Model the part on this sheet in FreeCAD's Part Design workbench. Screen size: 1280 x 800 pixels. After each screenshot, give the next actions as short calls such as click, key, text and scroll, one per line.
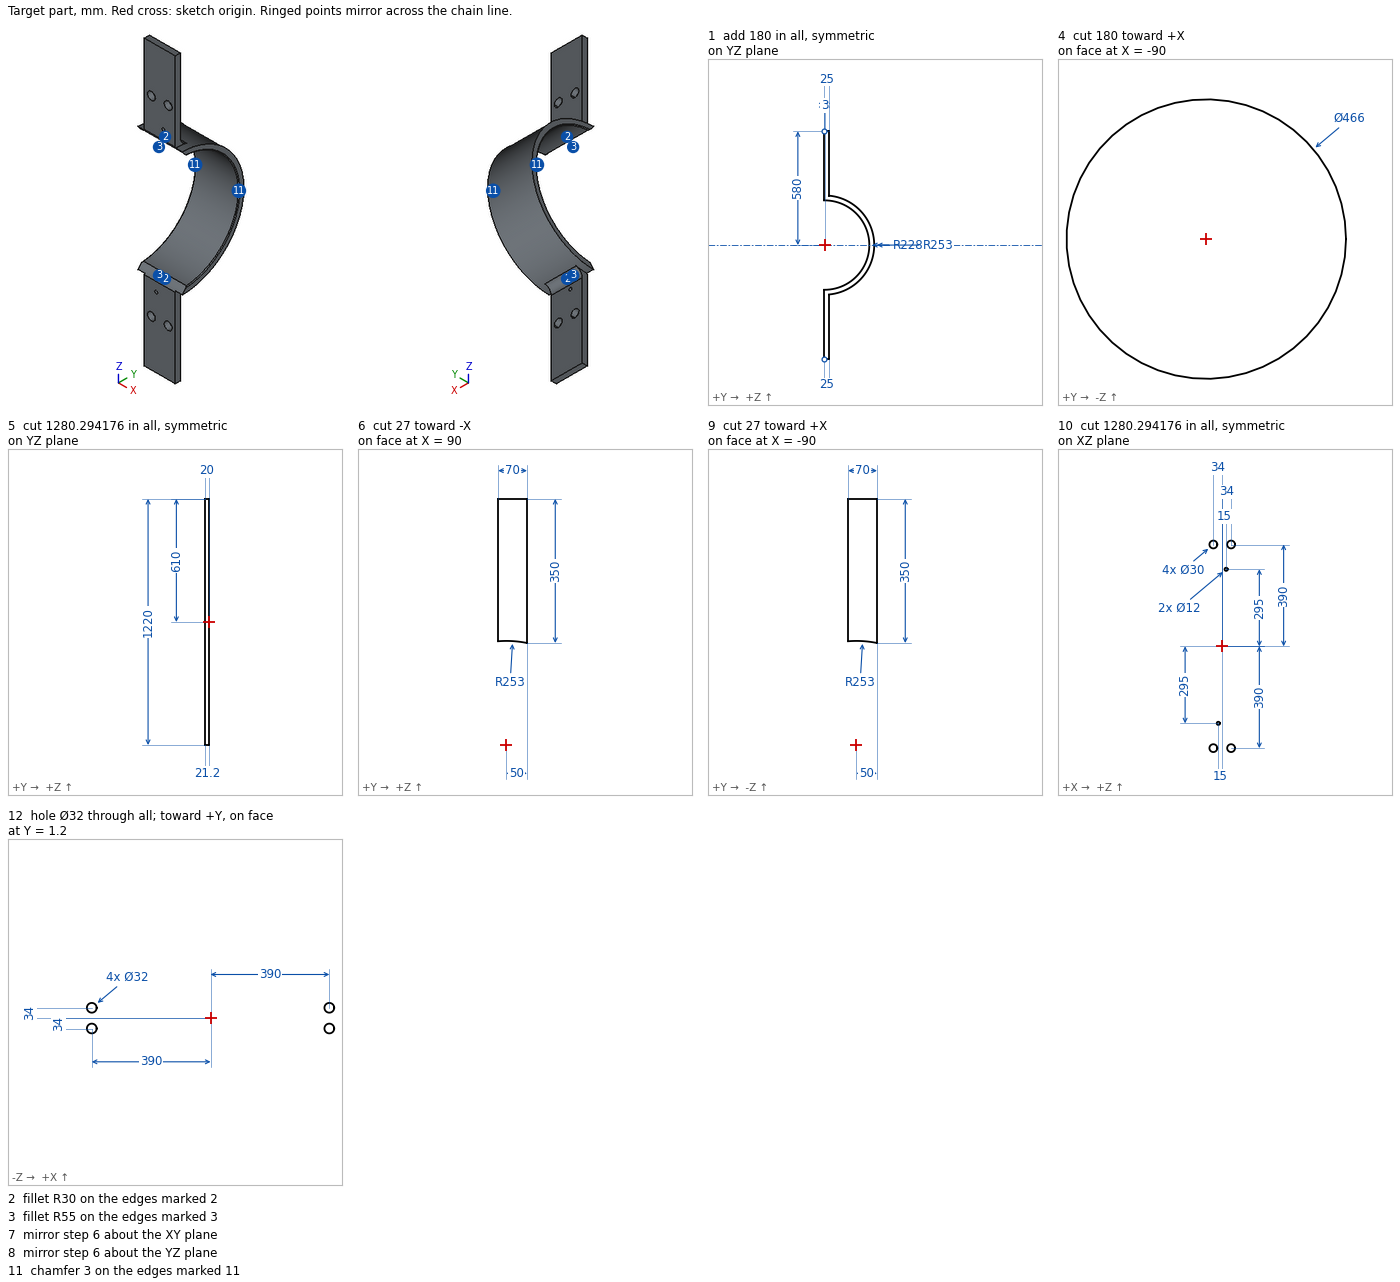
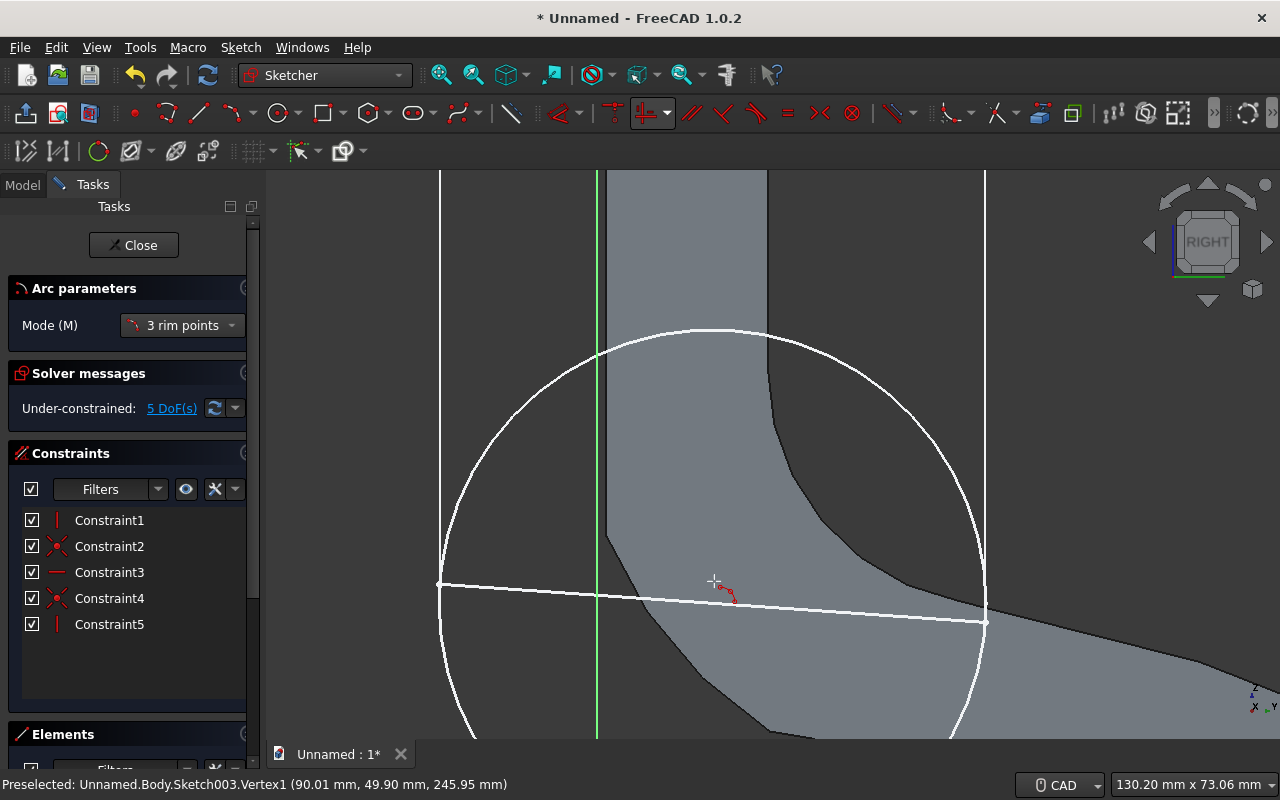
click(715, 571)
key(Escape)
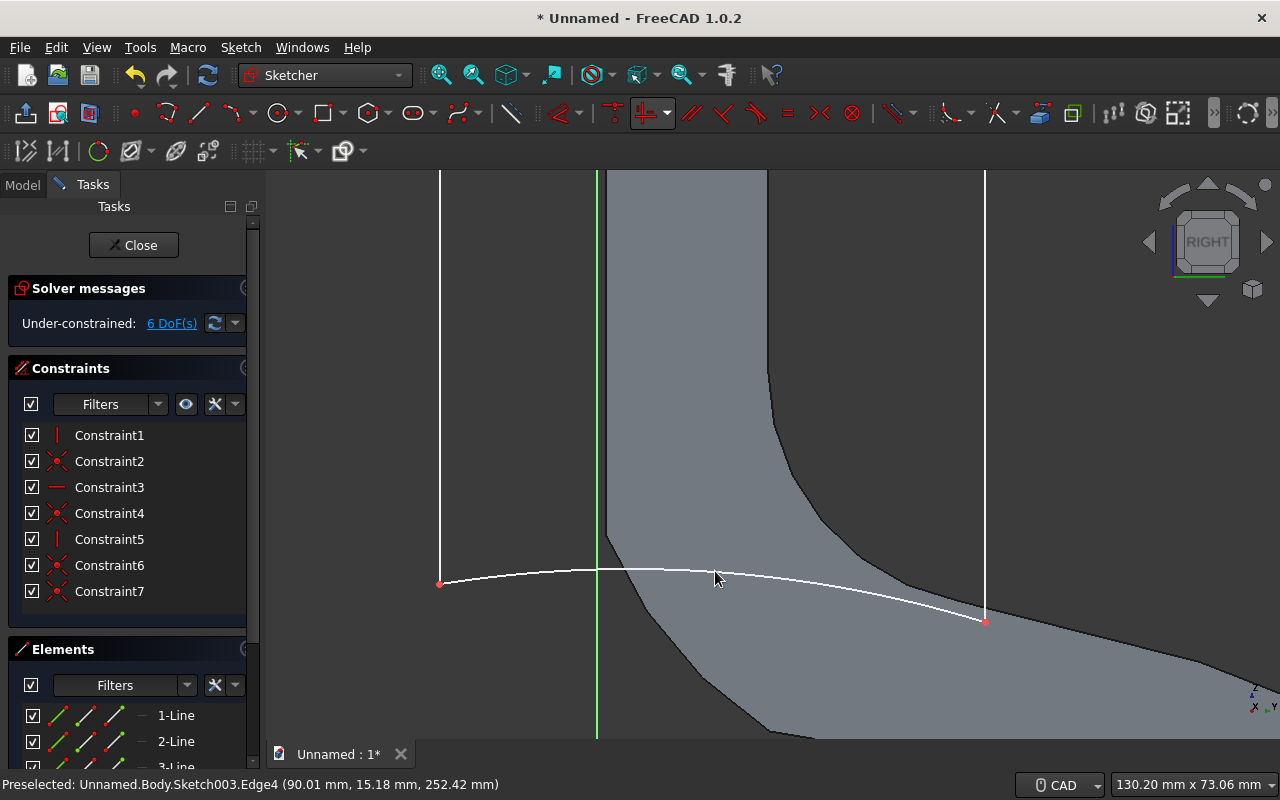
scroll(704, 474, down, 13)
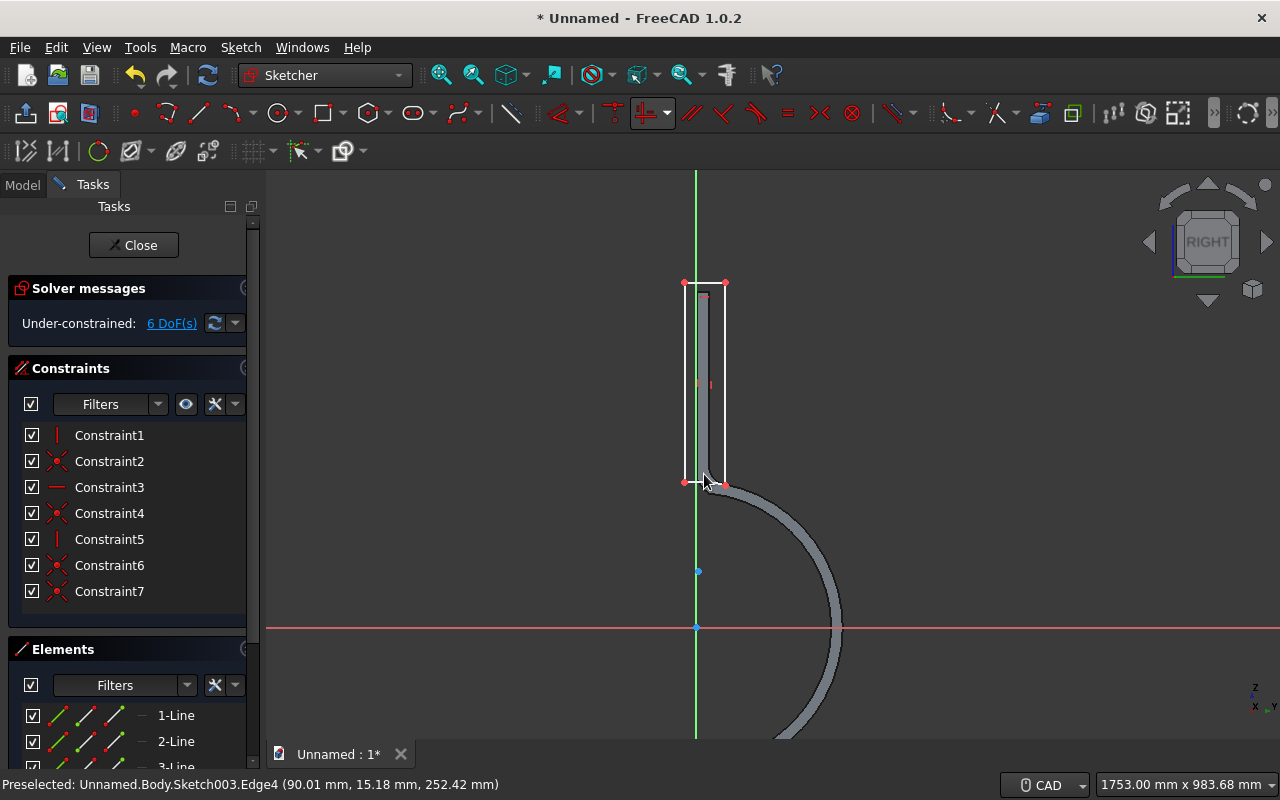
drag(686, 561, 709, 638)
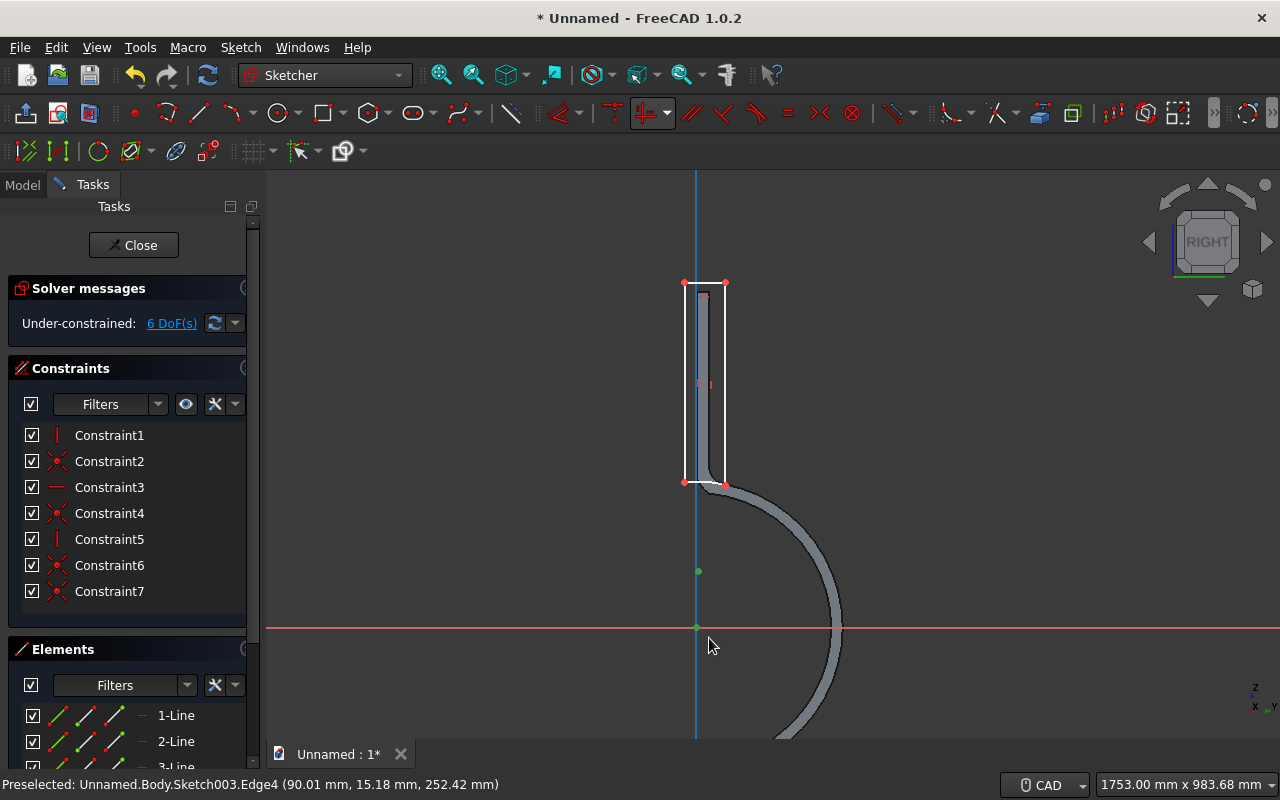
click(614, 114)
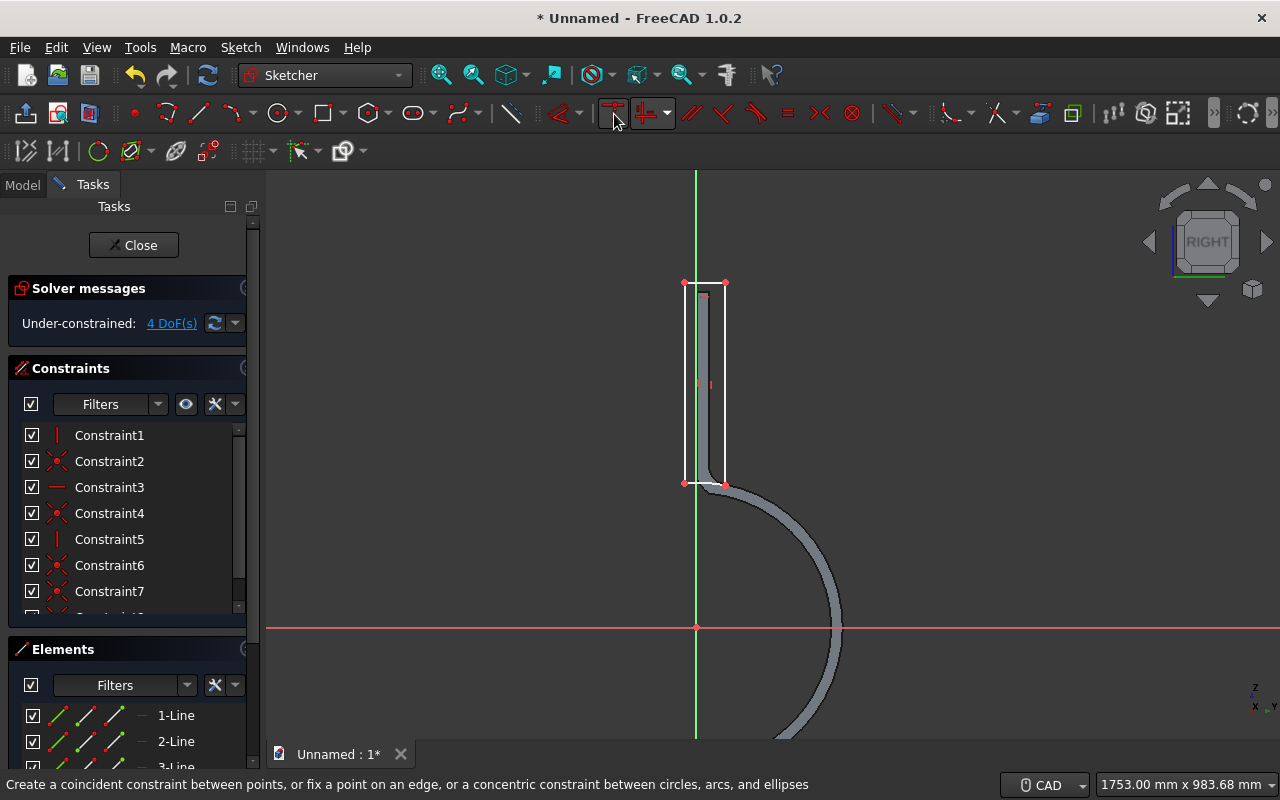
click(558, 114)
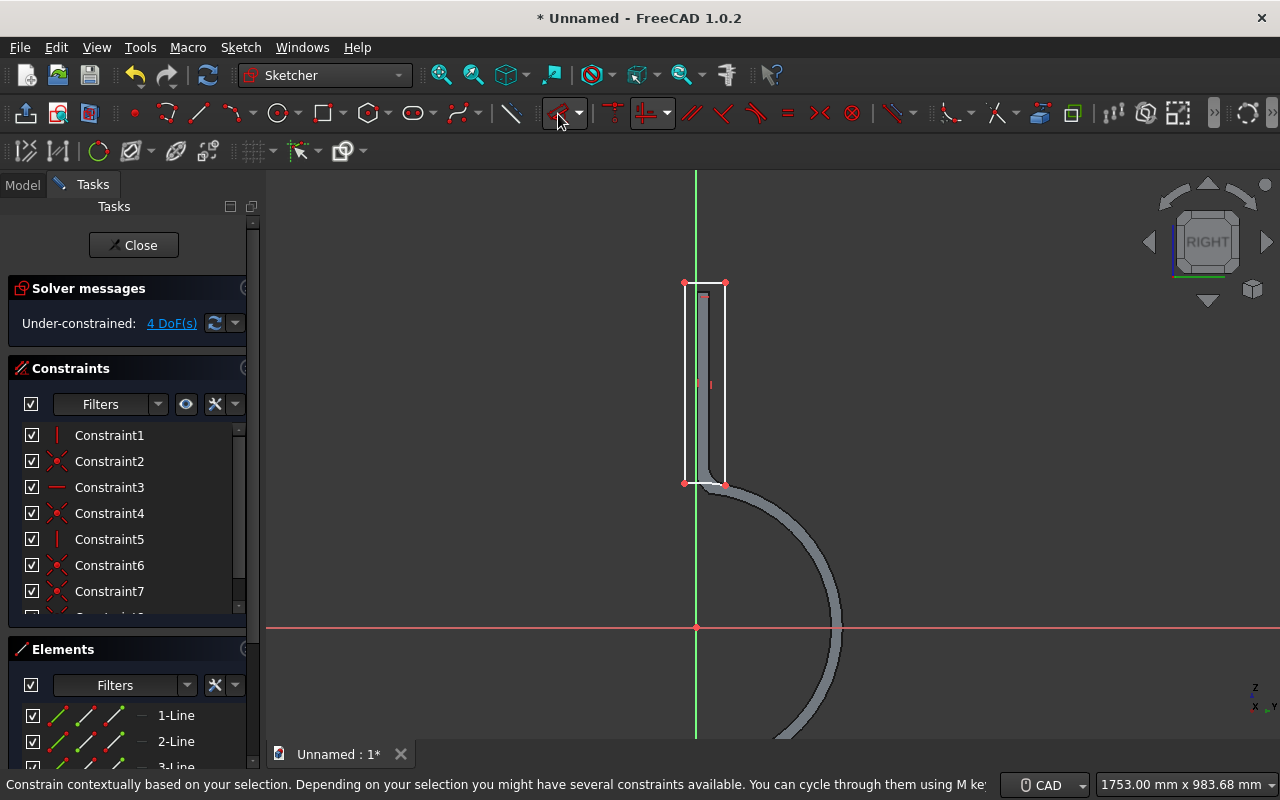
click(713, 484)
click(798, 483)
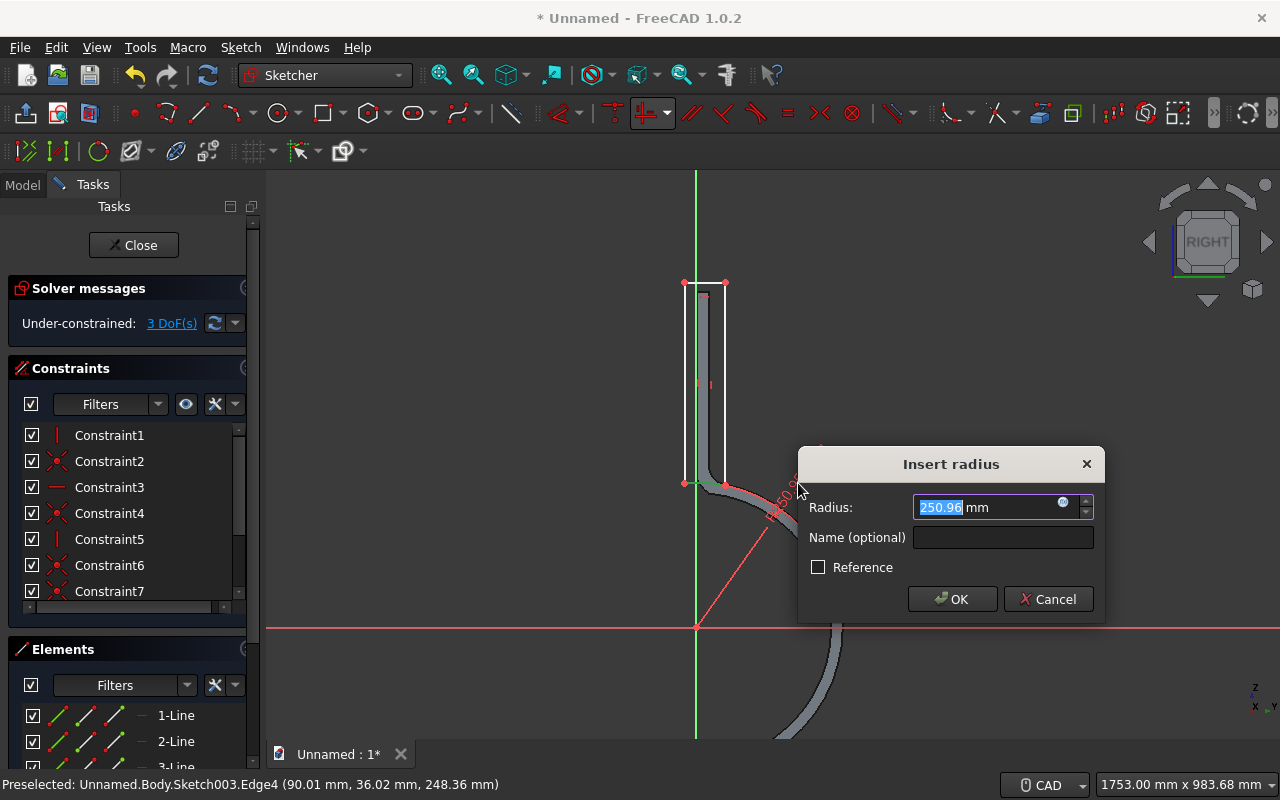
text(253)
key(Return)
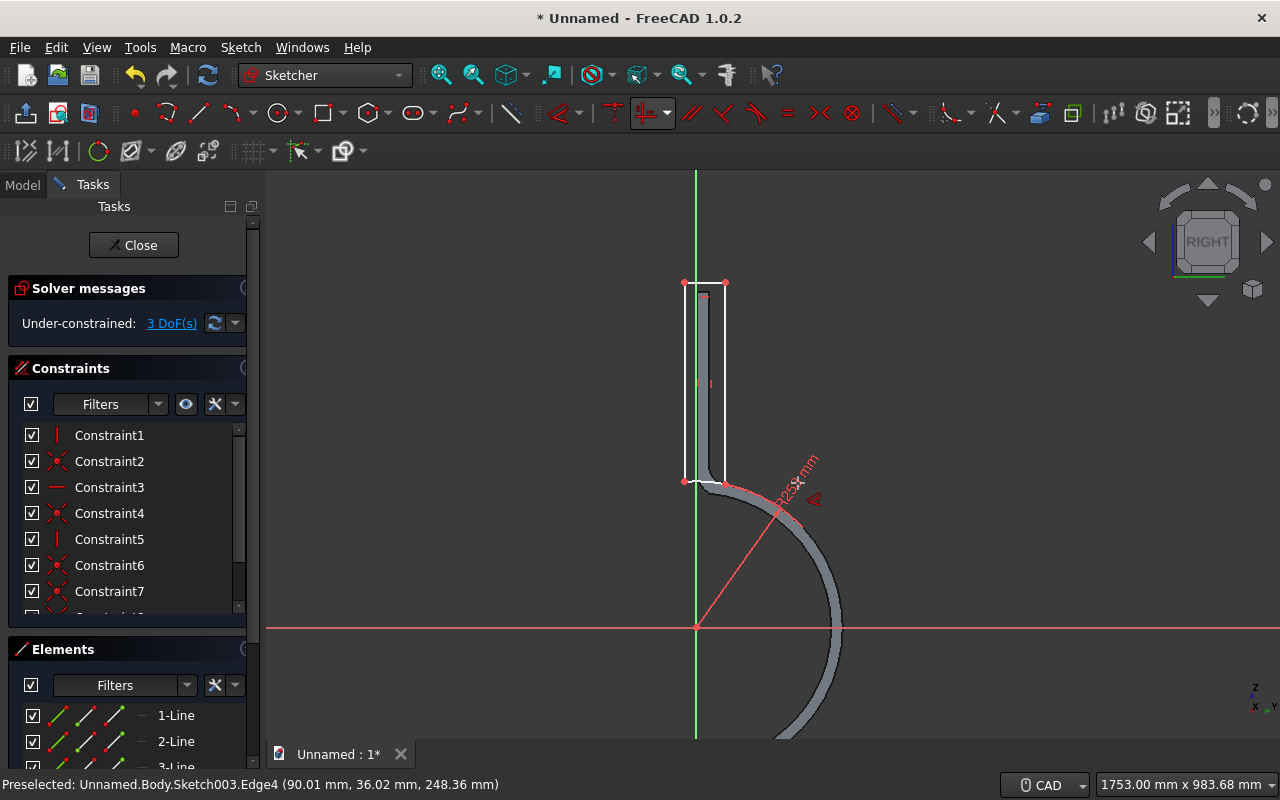
click(713, 283)
click(714, 249)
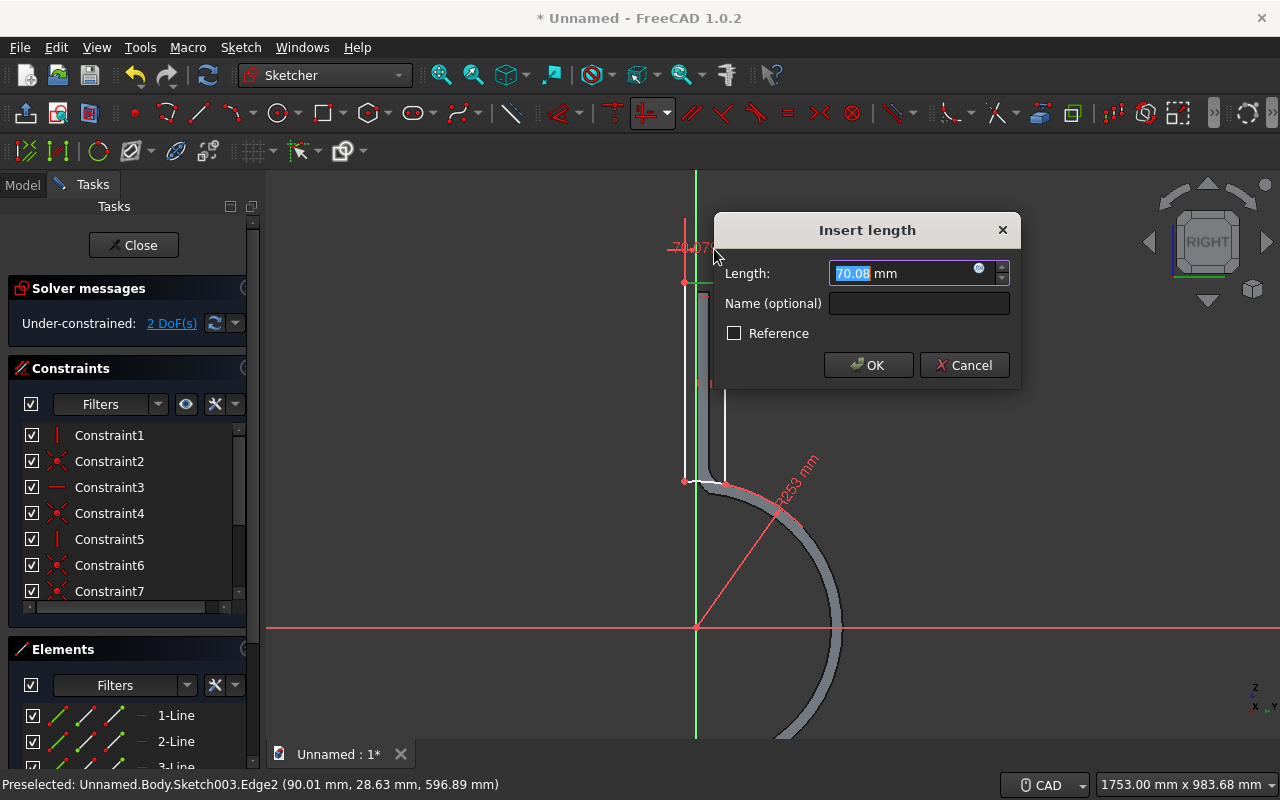
text(70)
key(Return)